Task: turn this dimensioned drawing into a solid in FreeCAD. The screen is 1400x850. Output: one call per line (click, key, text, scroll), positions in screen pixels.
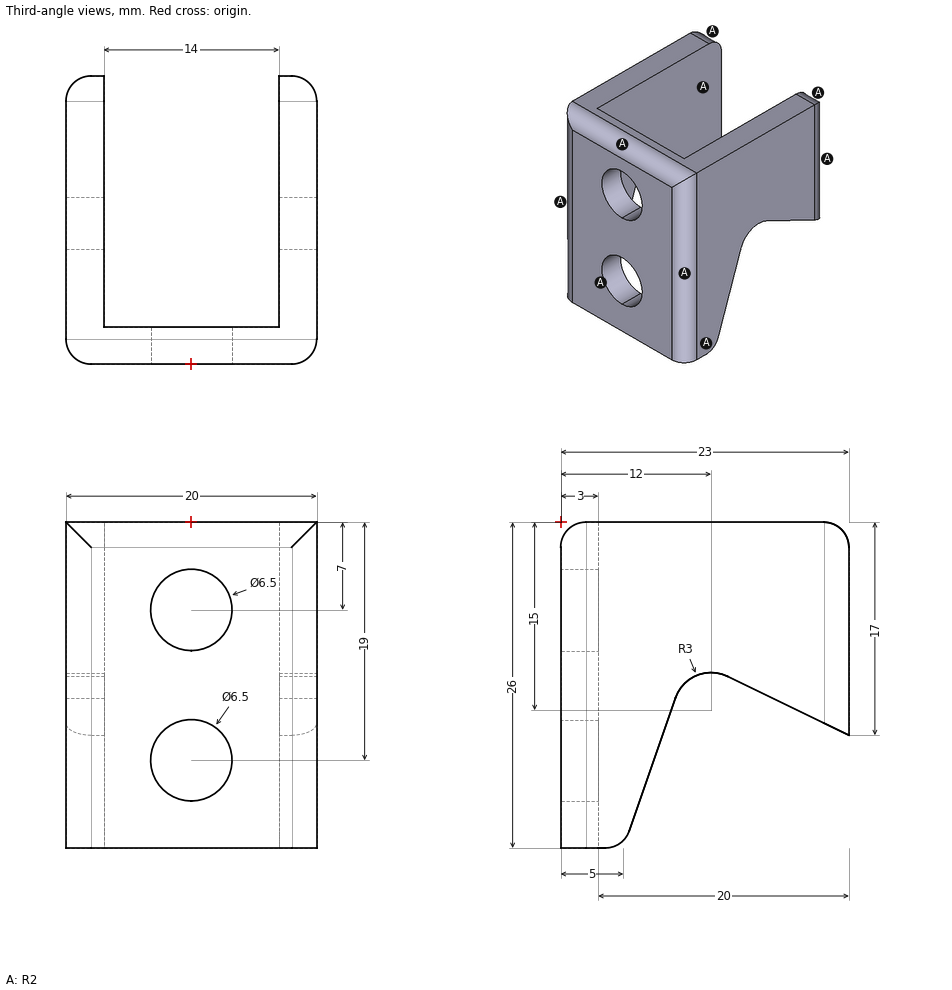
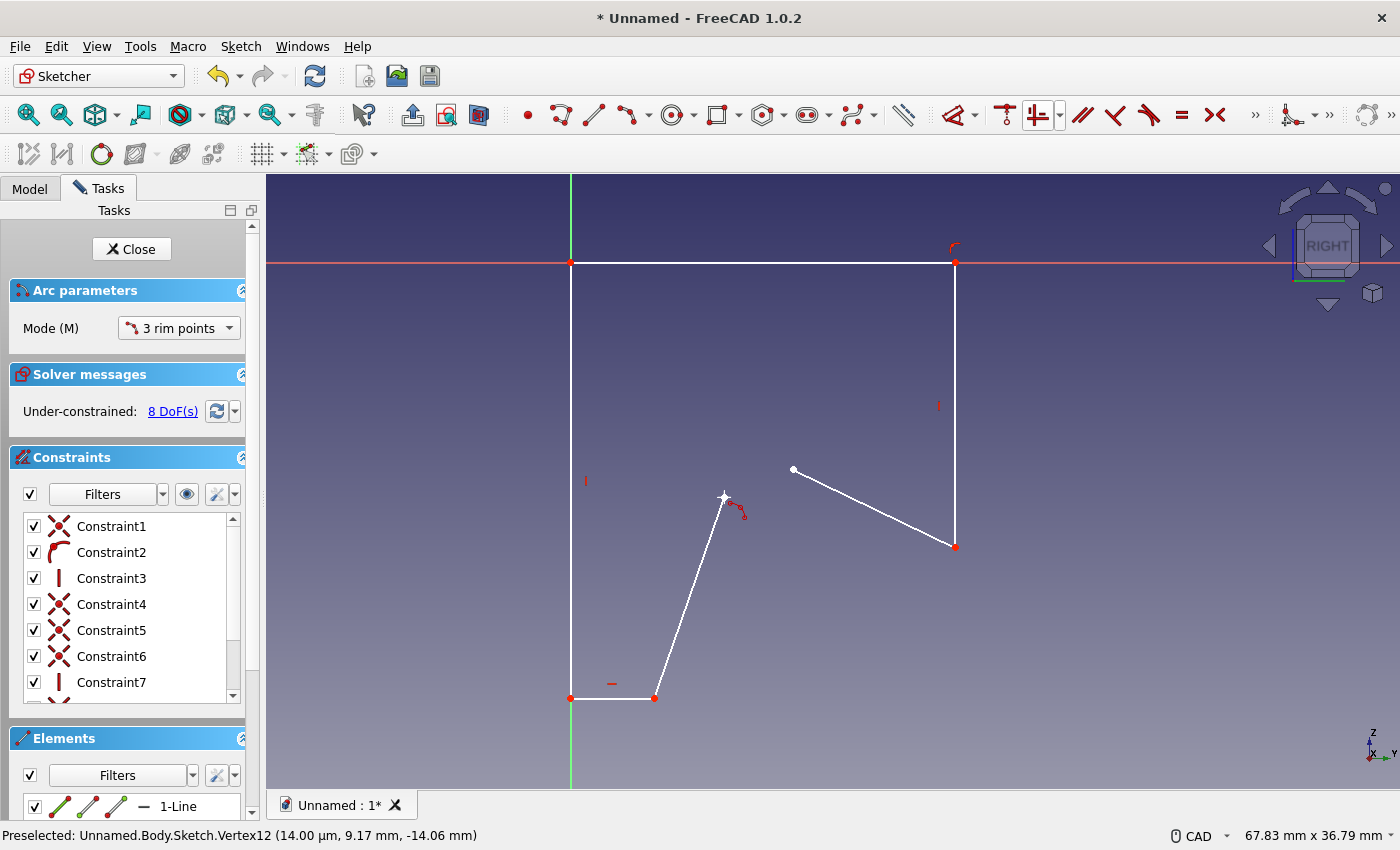
click(724, 498)
click(793, 470)
click(752, 467)
key(Escape)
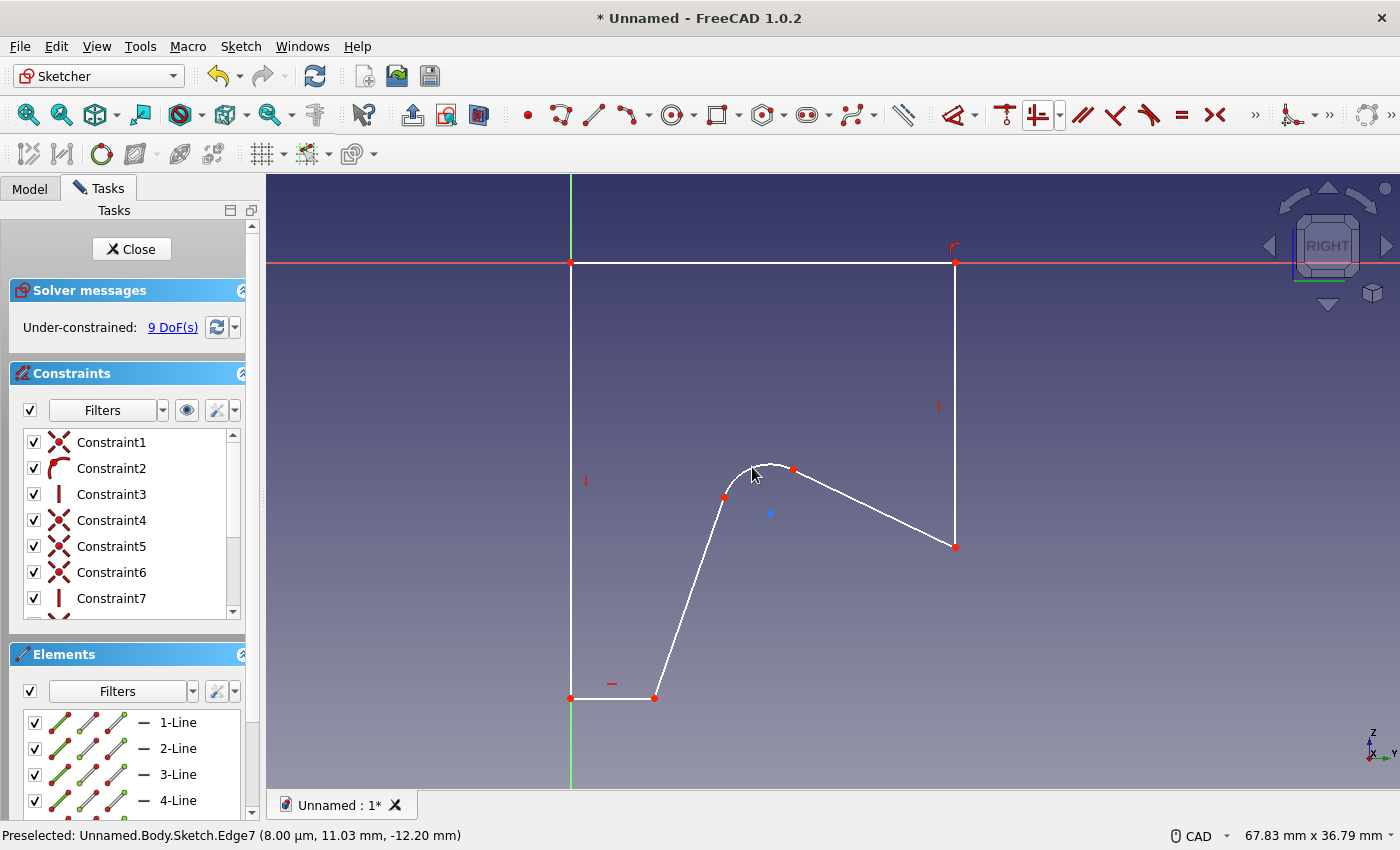
click(842, 493)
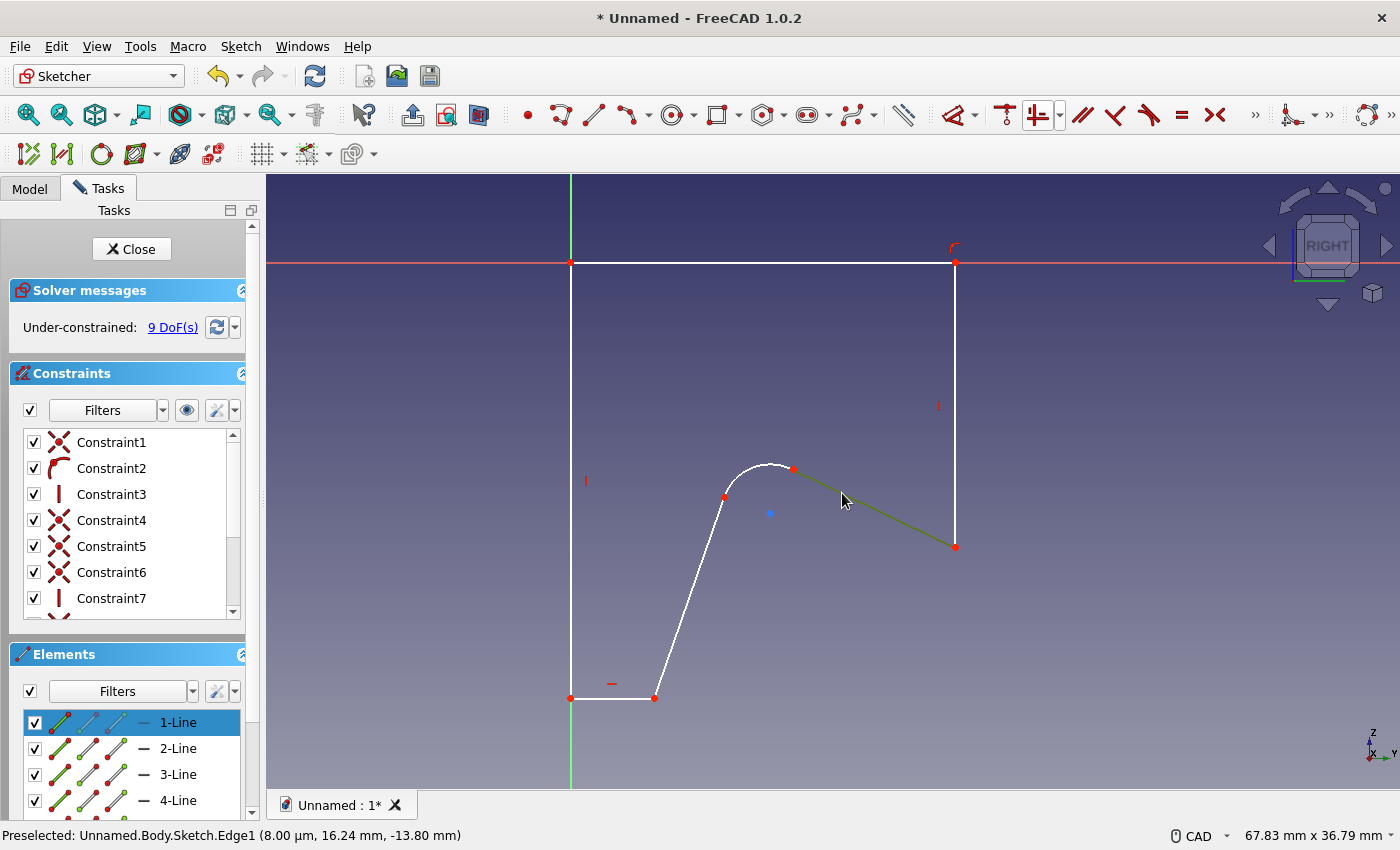
click(768, 464)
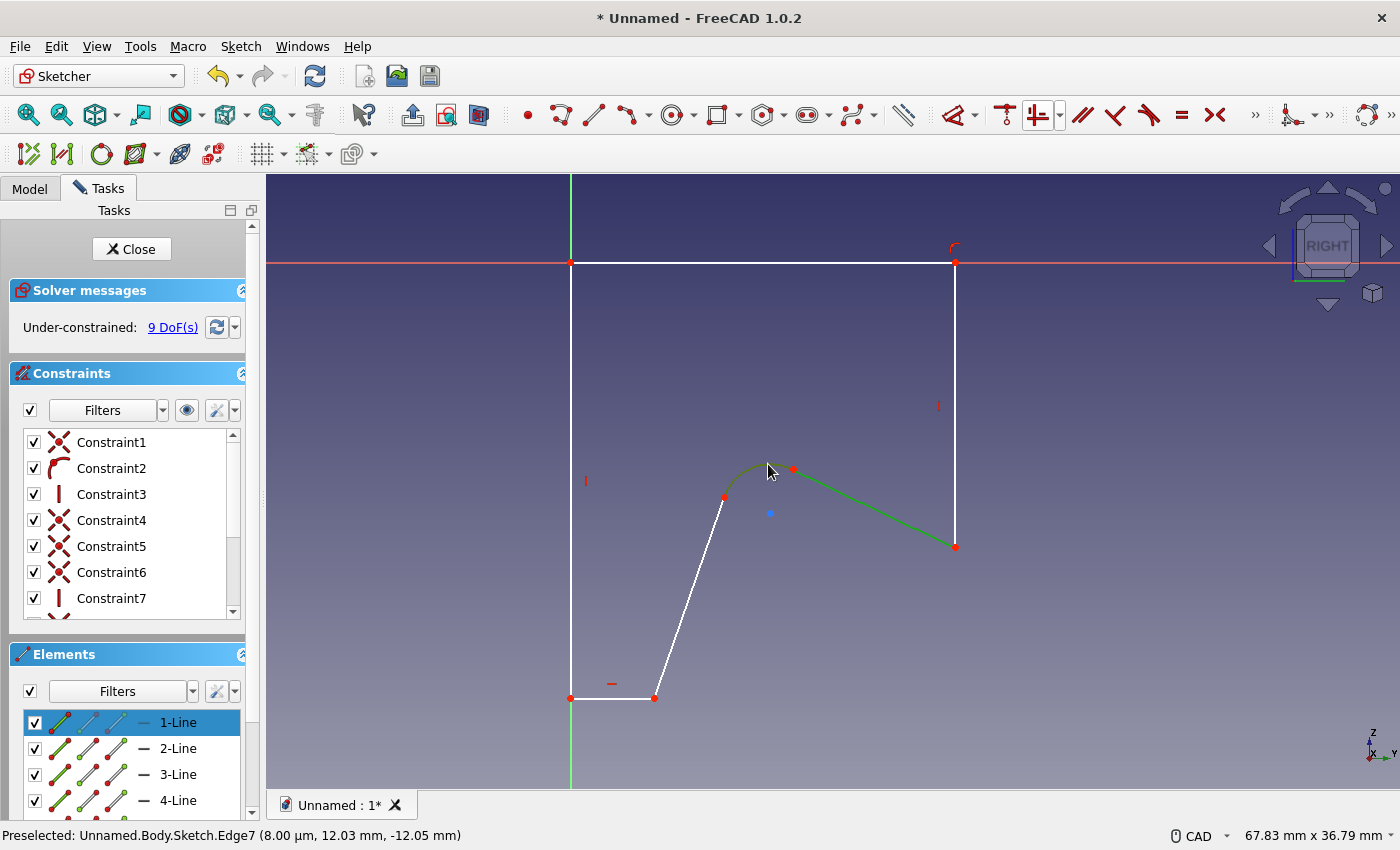
click(1149, 116)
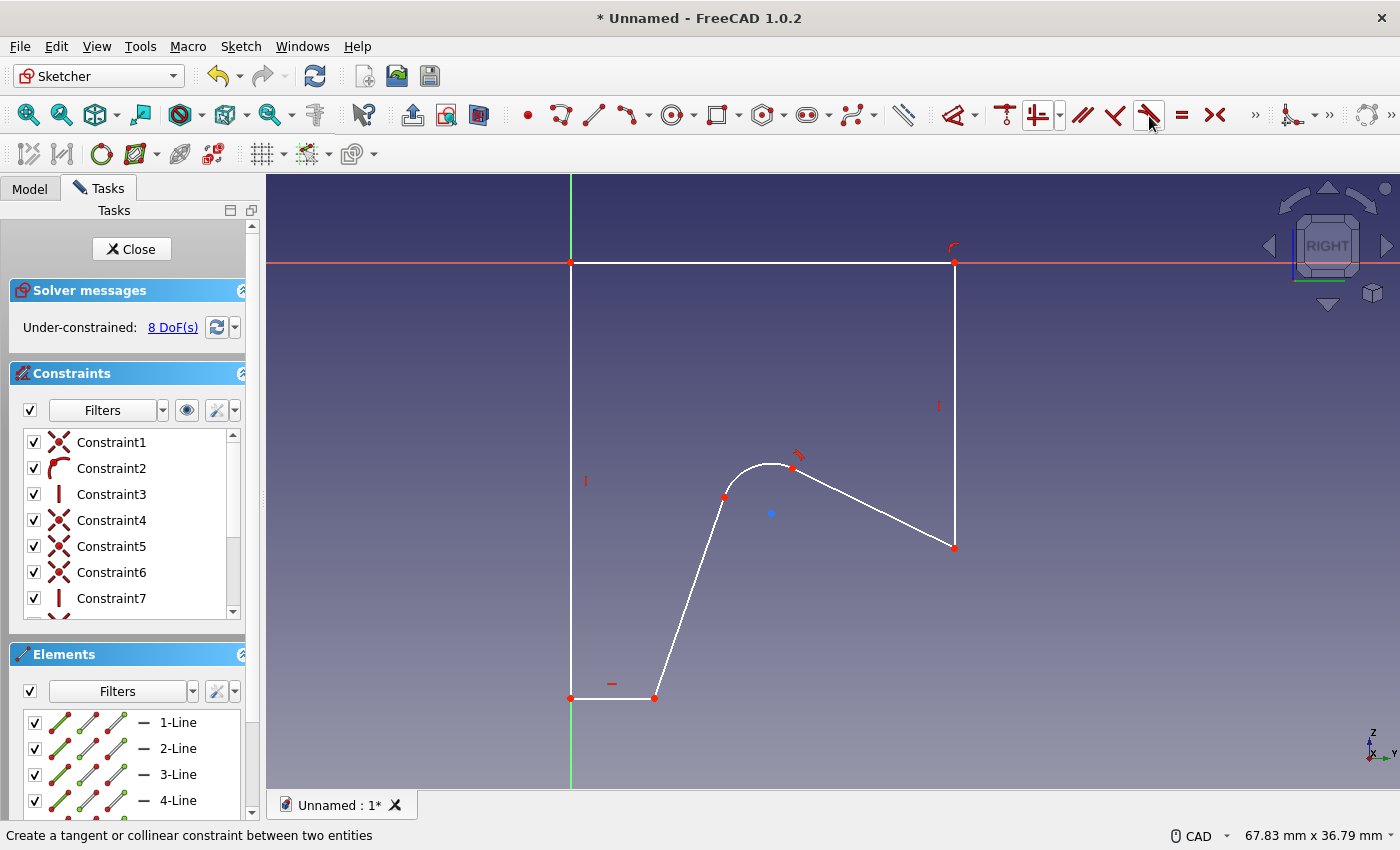
click(675, 639)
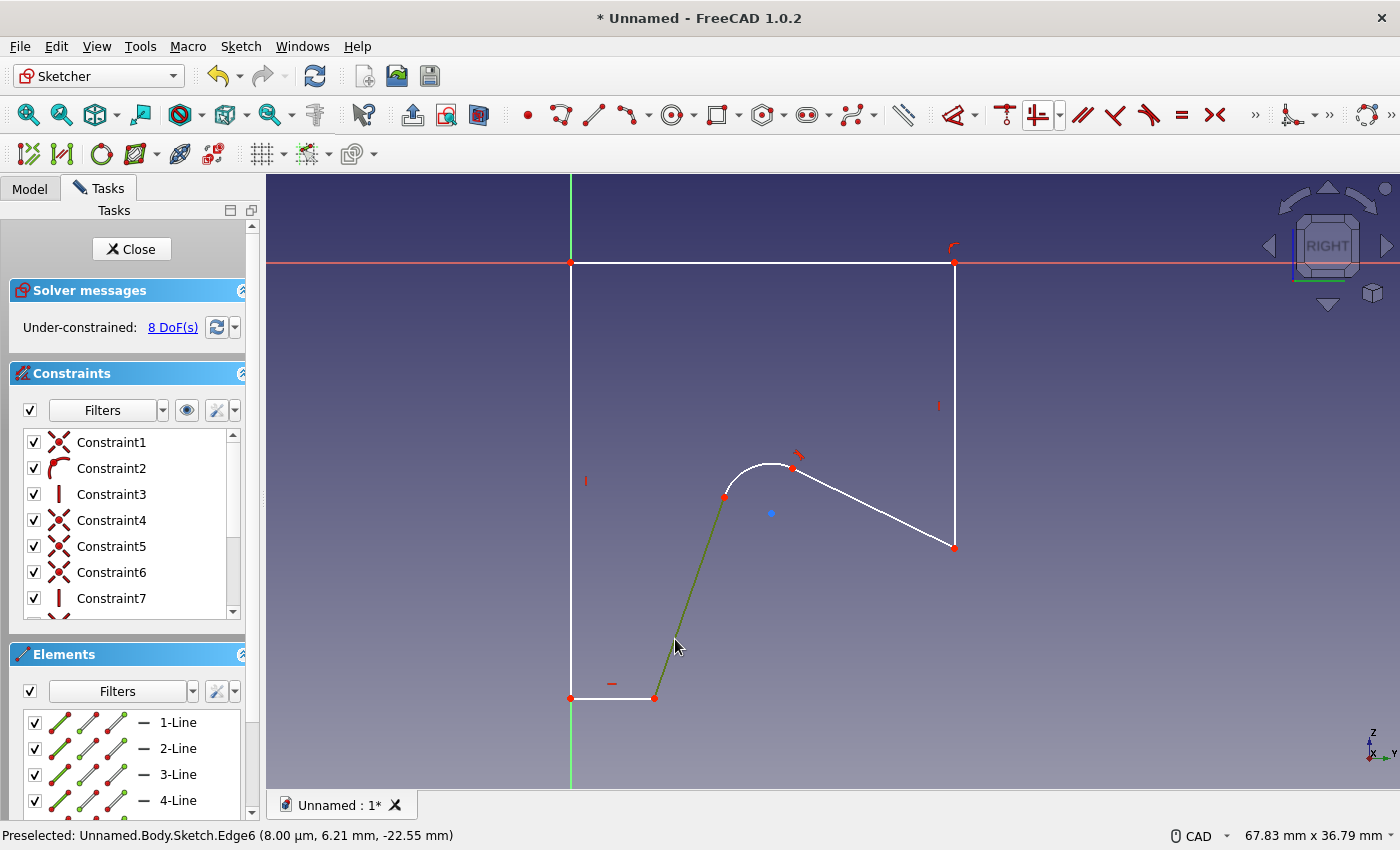
click(768, 464)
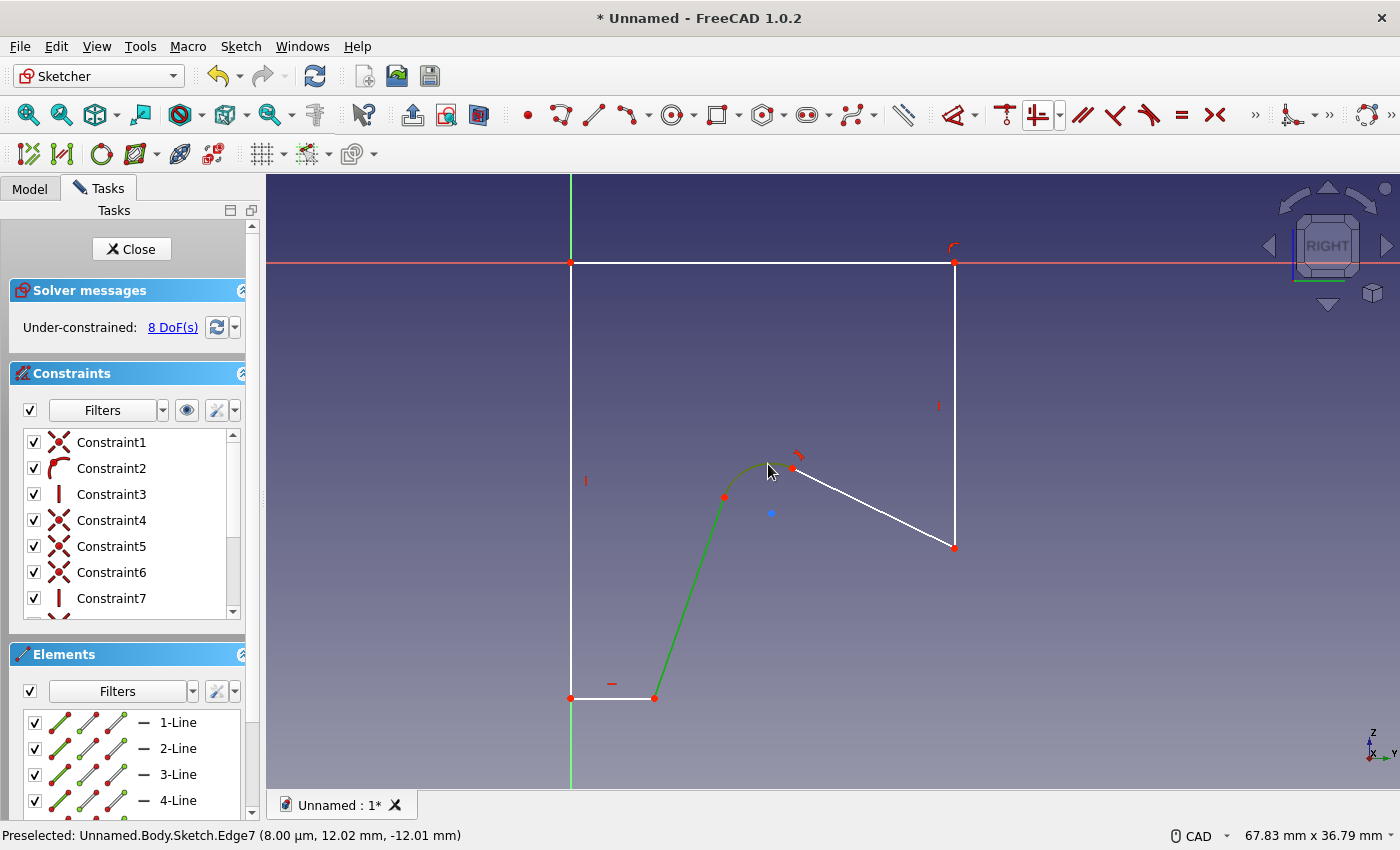
click(1149, 116)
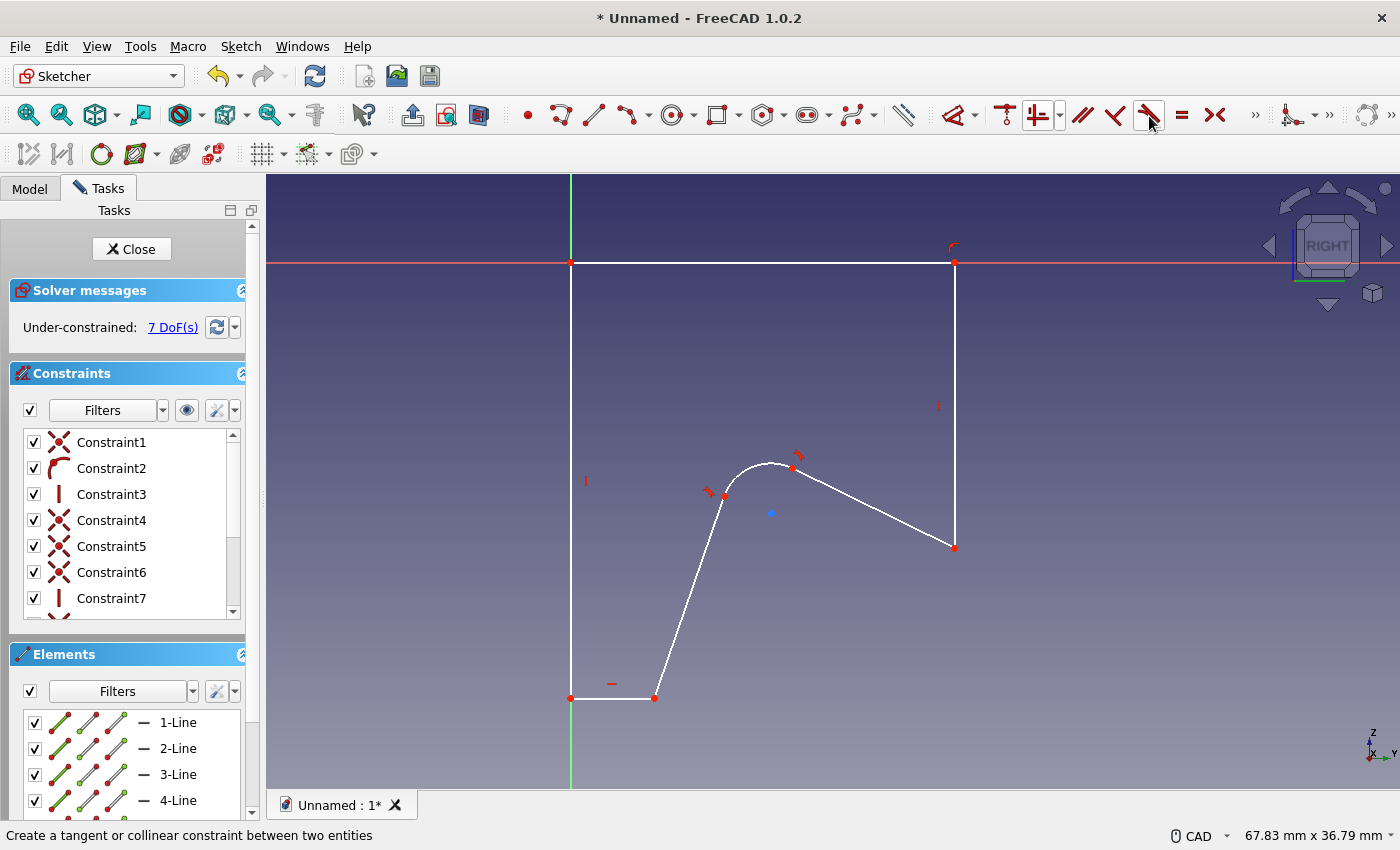
click(952, 116)